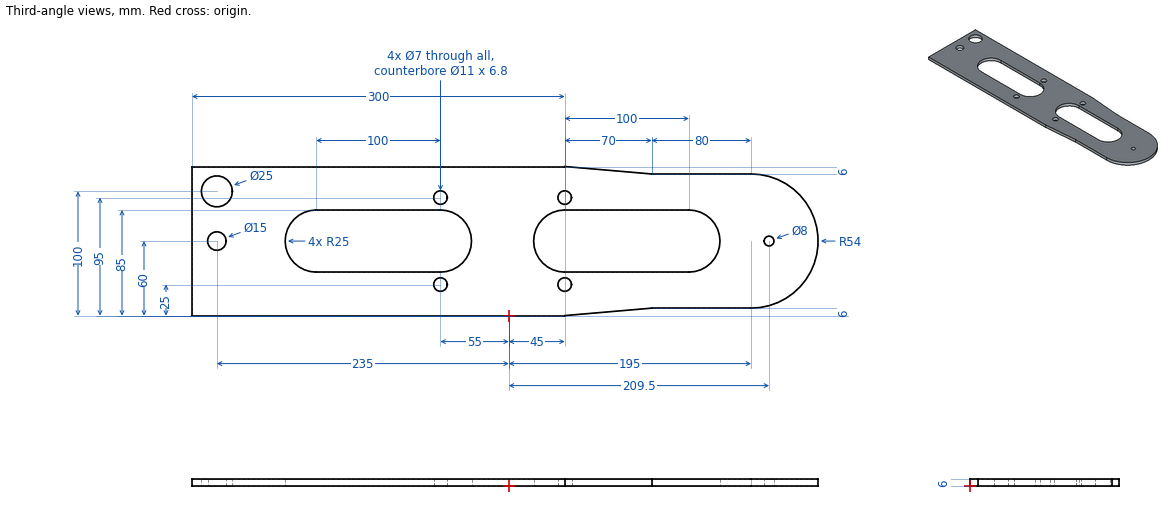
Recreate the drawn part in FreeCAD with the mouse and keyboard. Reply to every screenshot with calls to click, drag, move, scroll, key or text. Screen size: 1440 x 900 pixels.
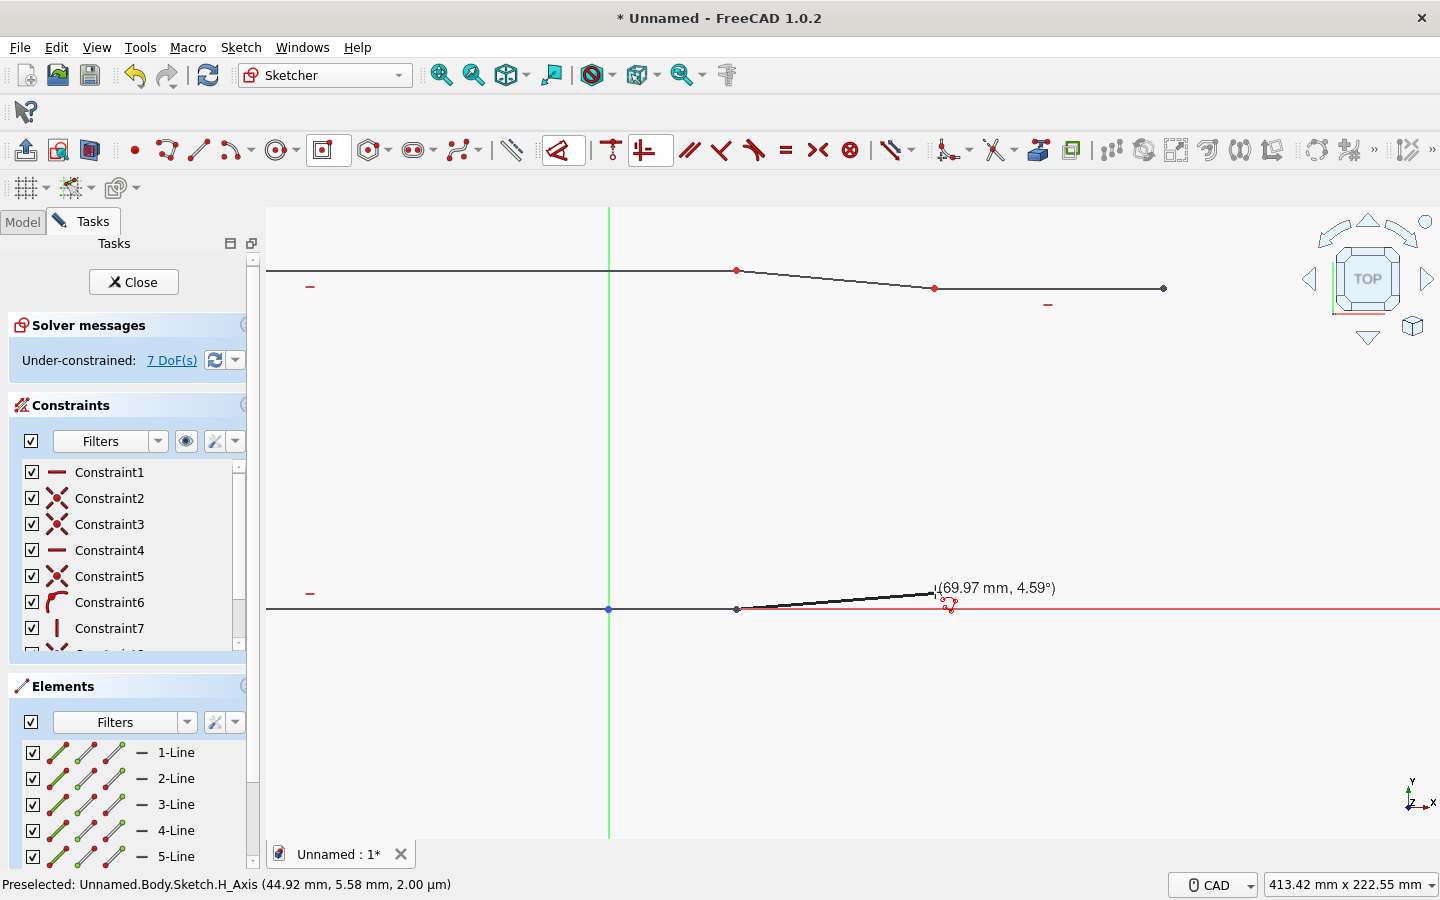
click(935, 592)
click(1162, 592)
right_click(1162, 592)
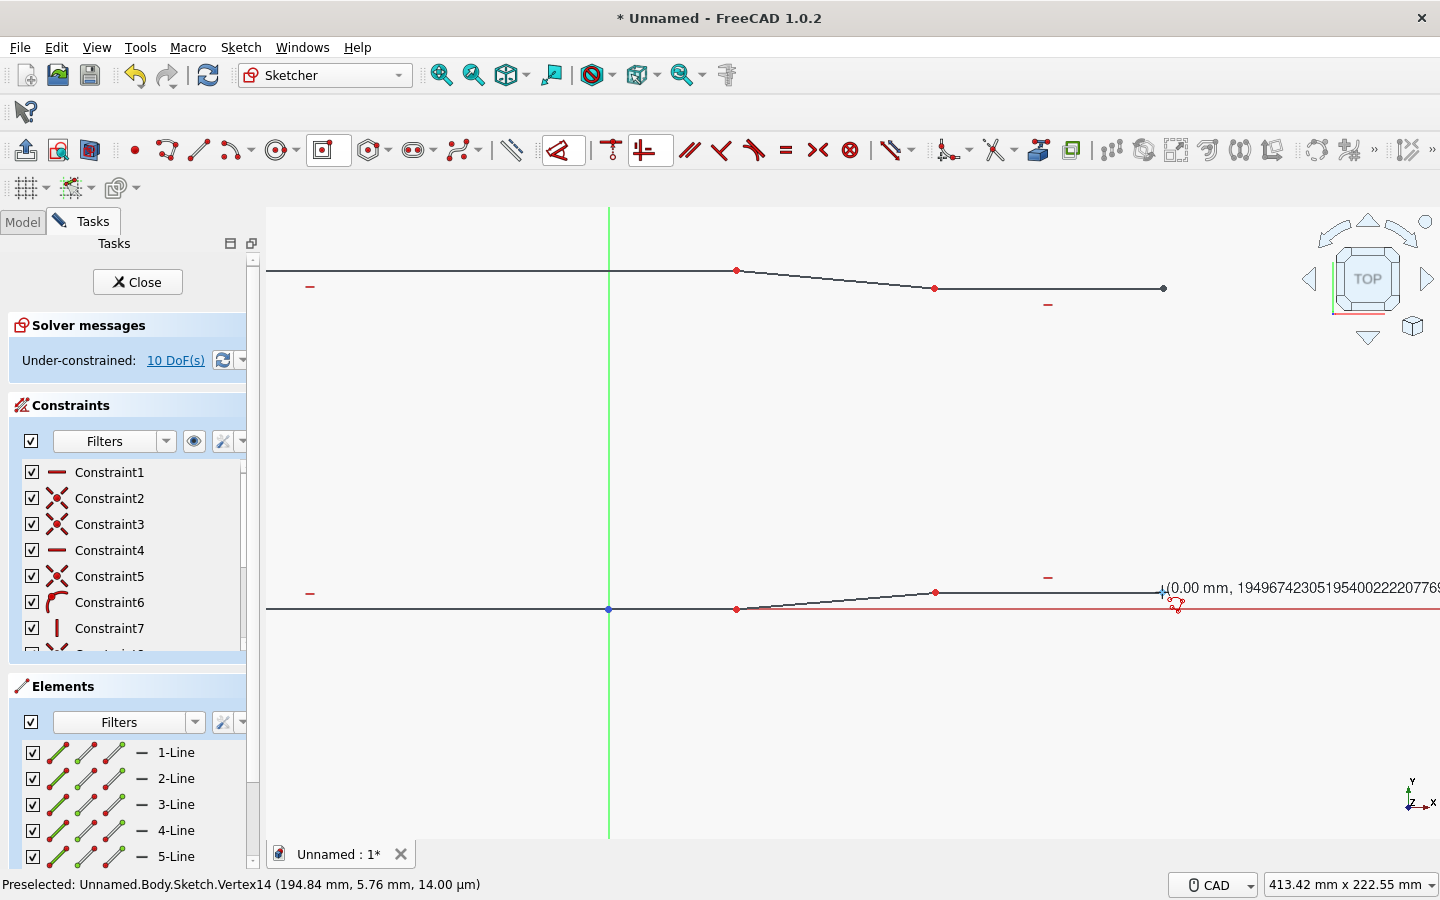
click(254, 150)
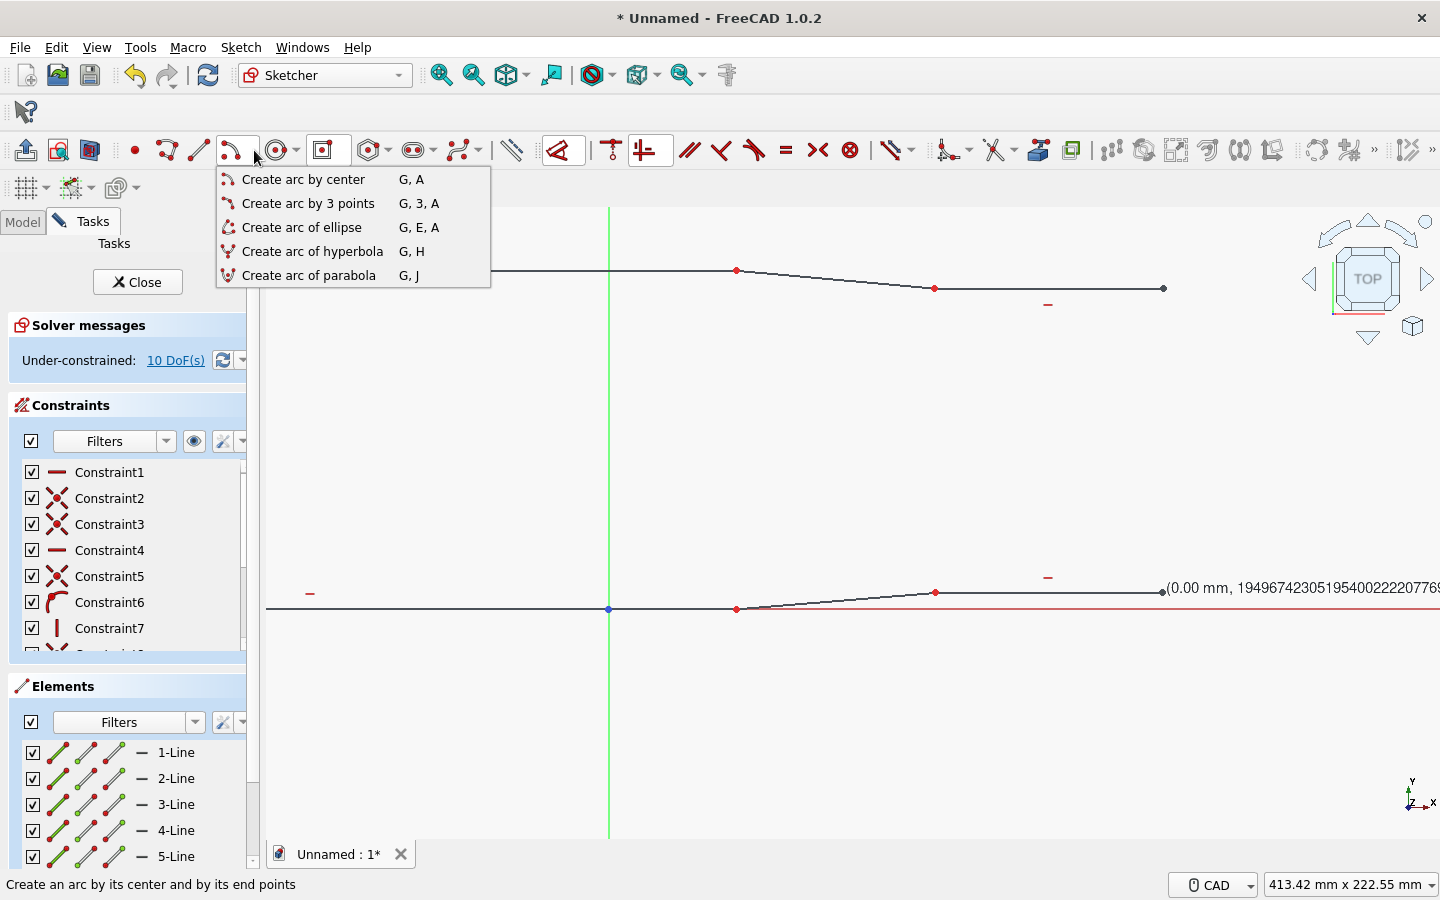
click(354, 203)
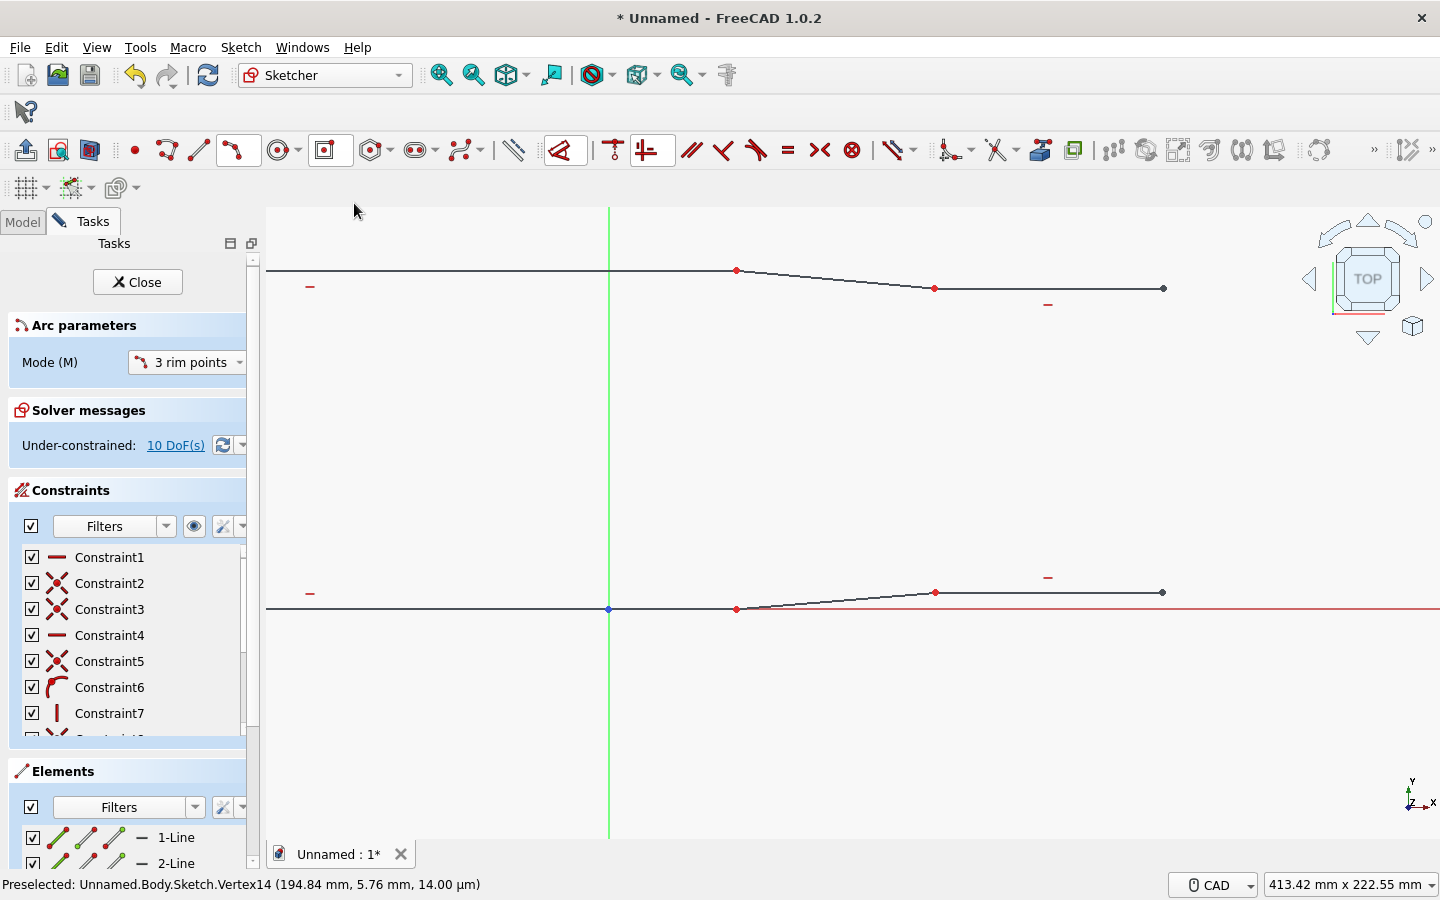
click(1162, 593)
click(1164, 289)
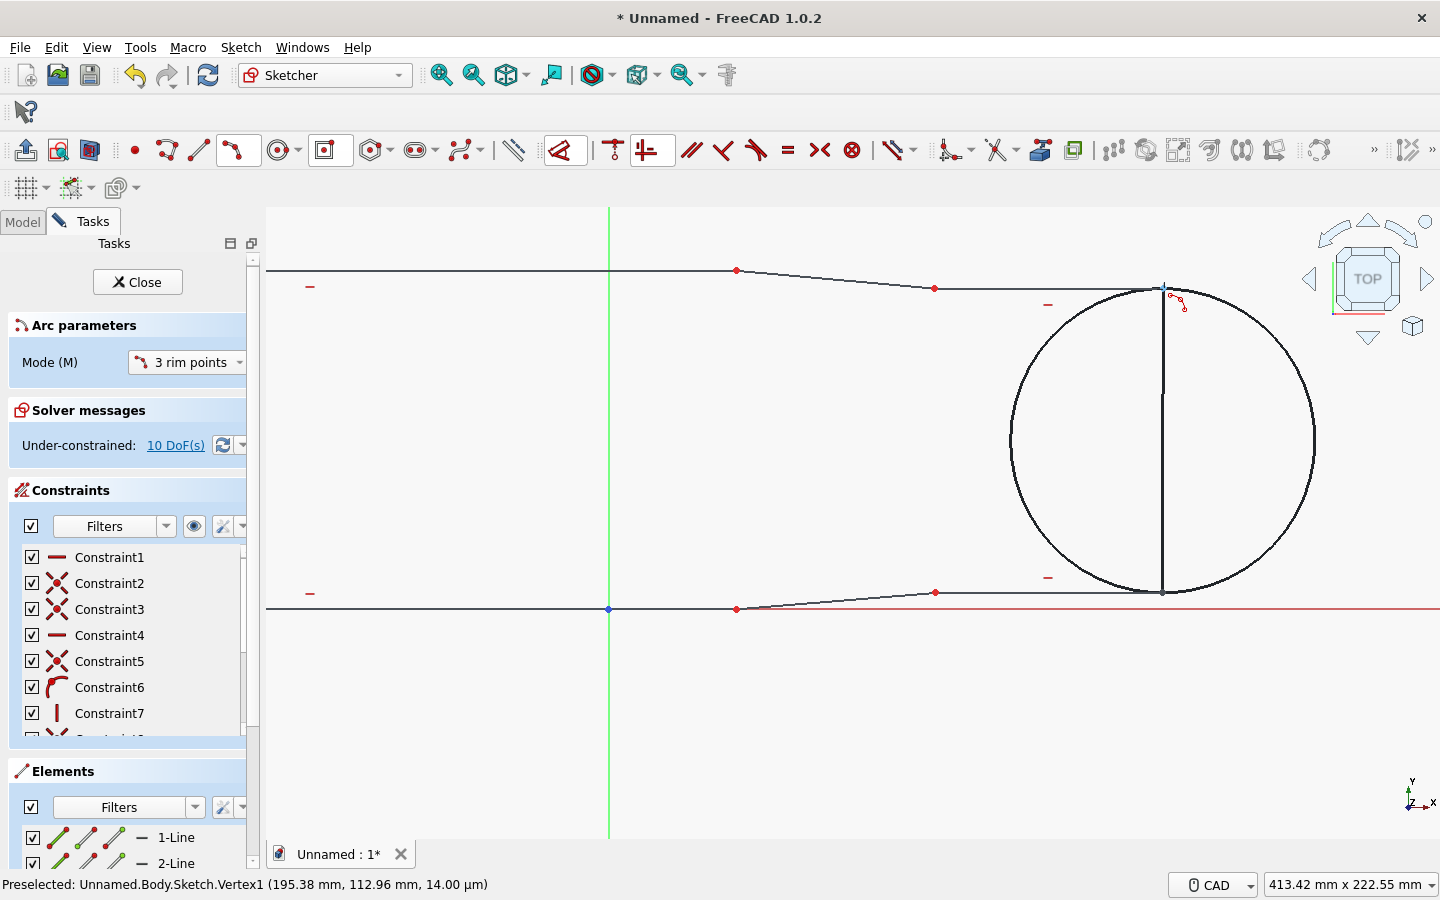
scroll(935, 592, down, 4)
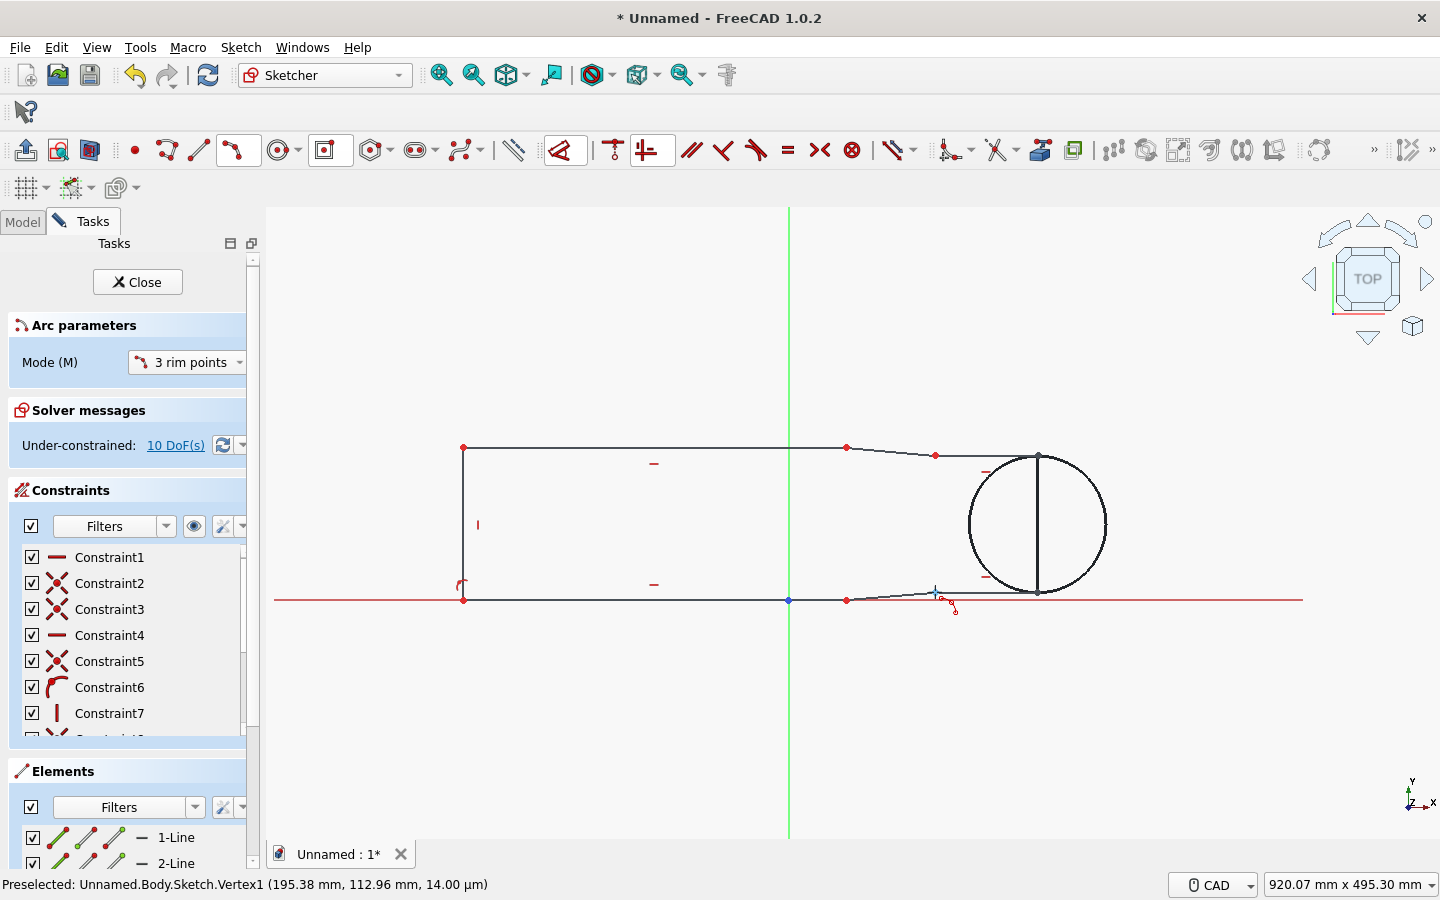
click(1106, 524)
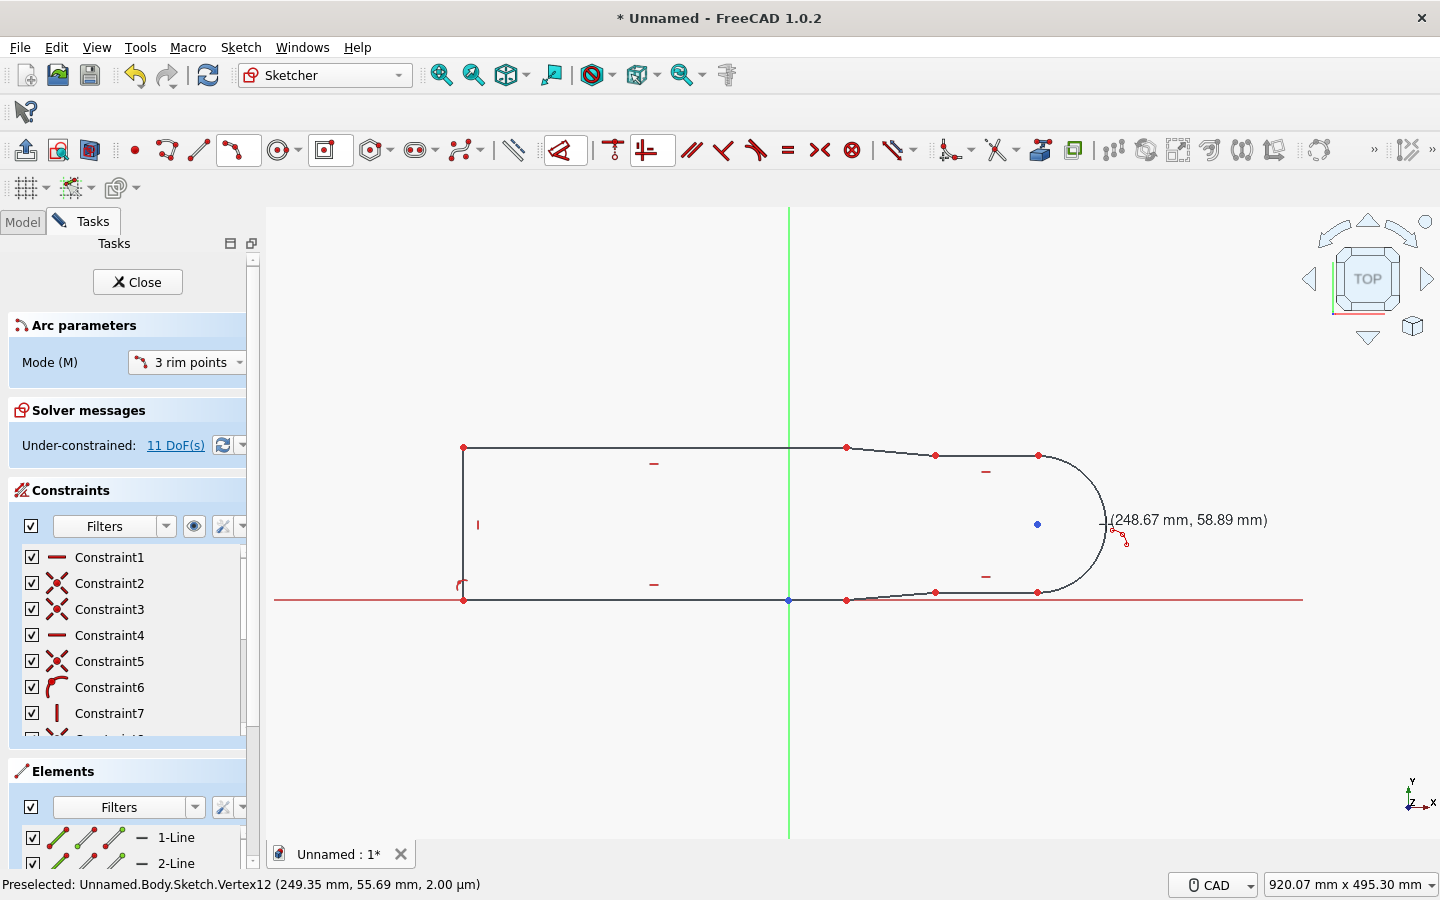
click(416, 150)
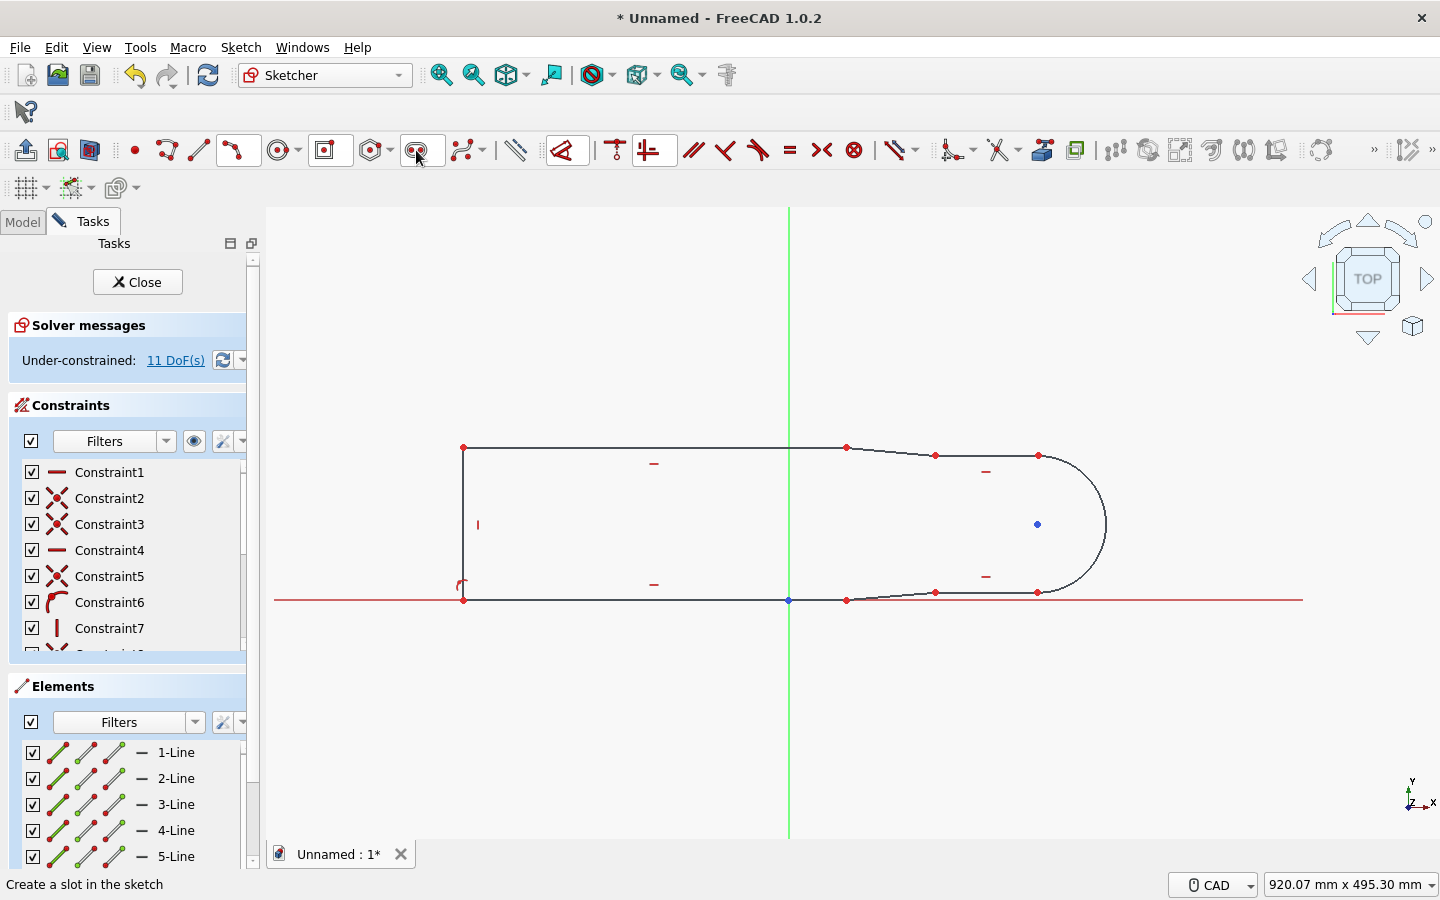
click(591, 524)